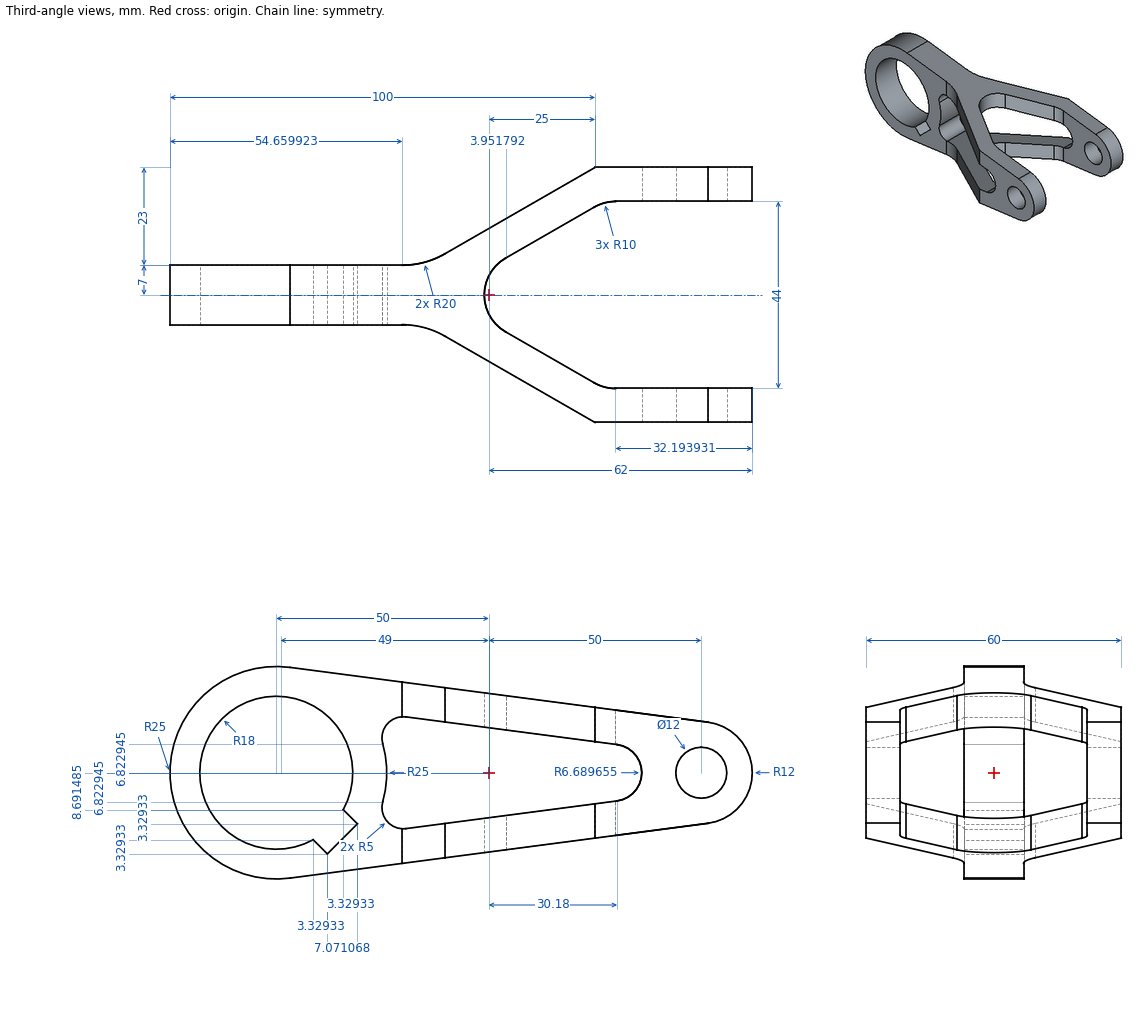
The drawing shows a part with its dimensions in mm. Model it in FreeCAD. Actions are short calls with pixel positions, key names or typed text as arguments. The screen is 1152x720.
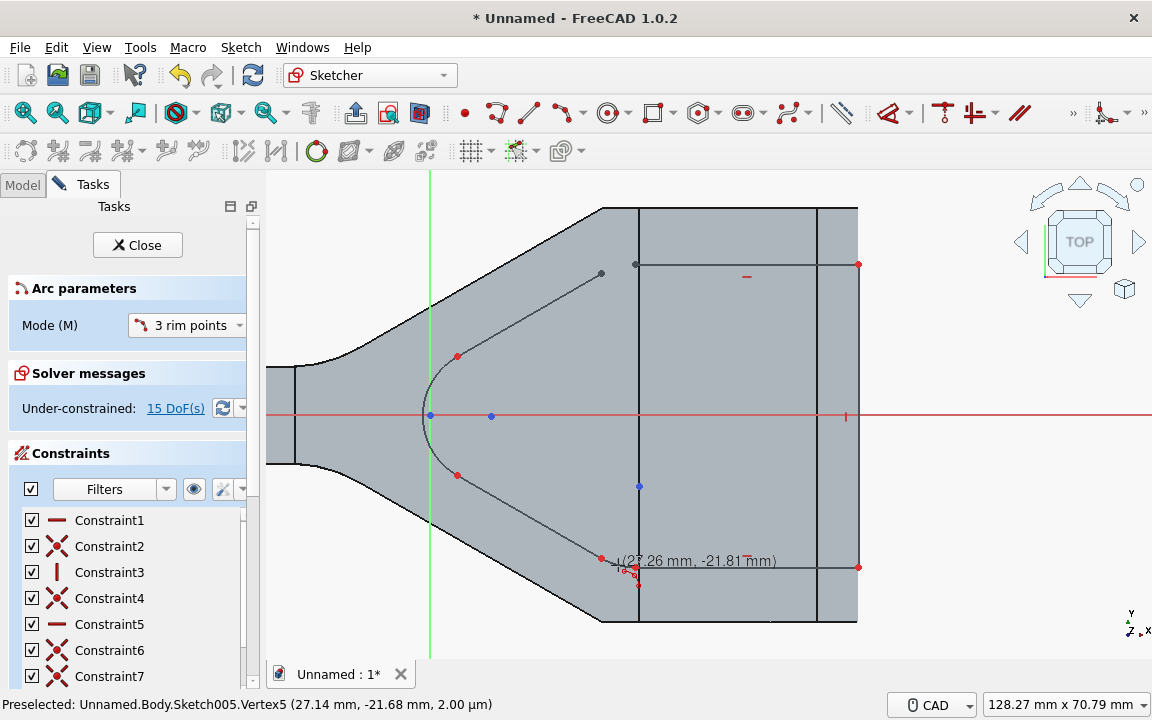
click(636, 265)
click(602, 274)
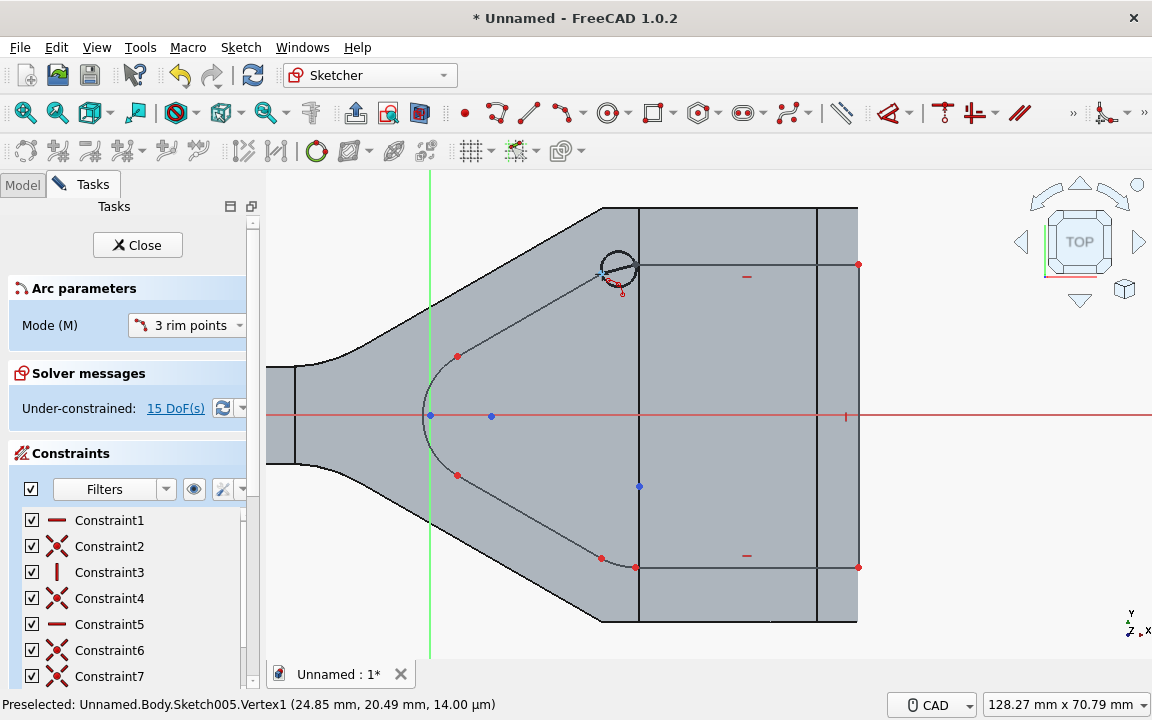
scroll(618, 266, up, 10)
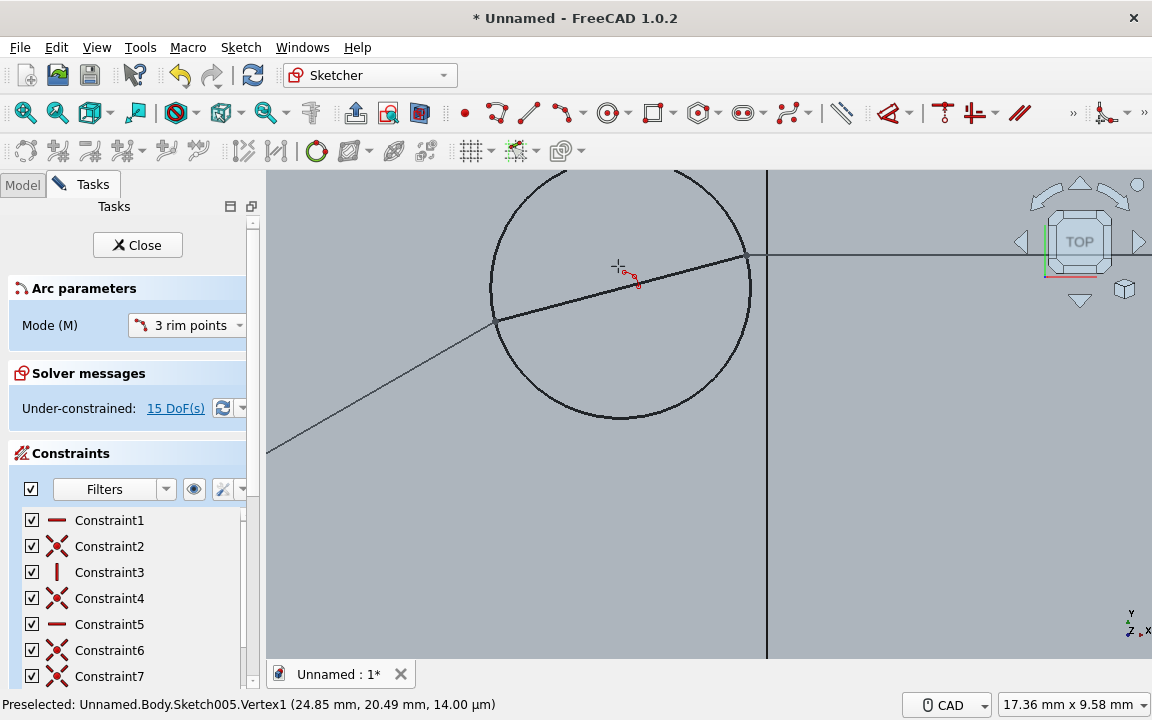
click(616, 262)
key(Escape)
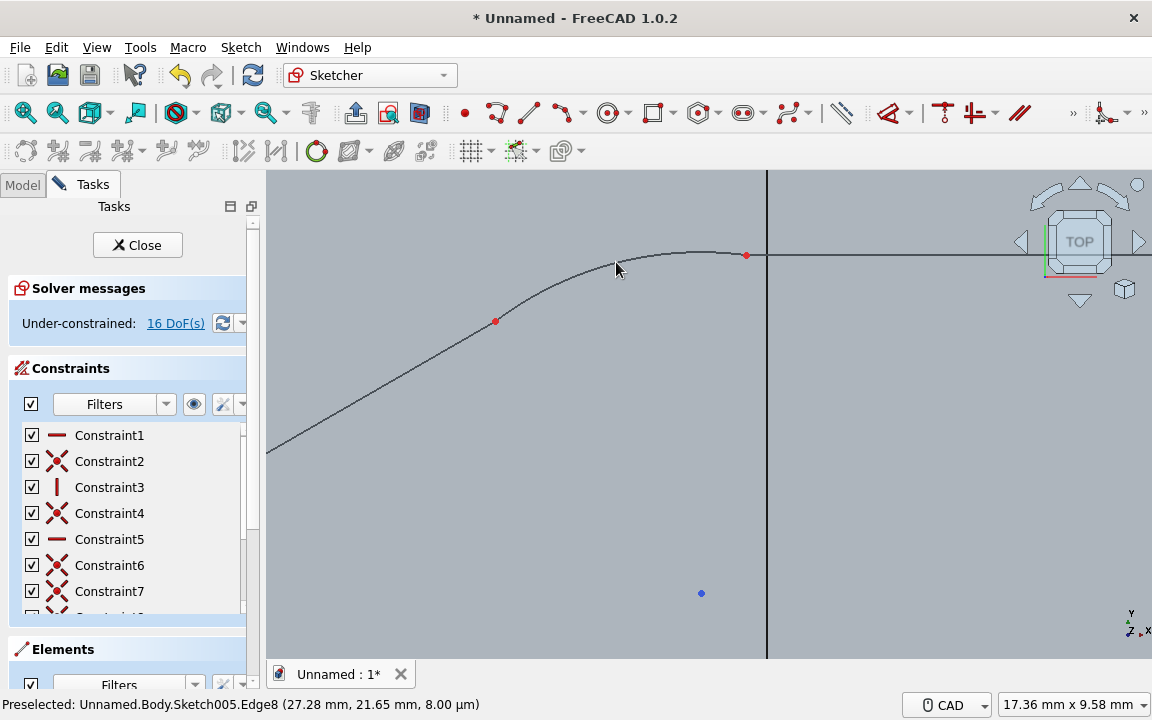
scroll(618, 265, down, 10)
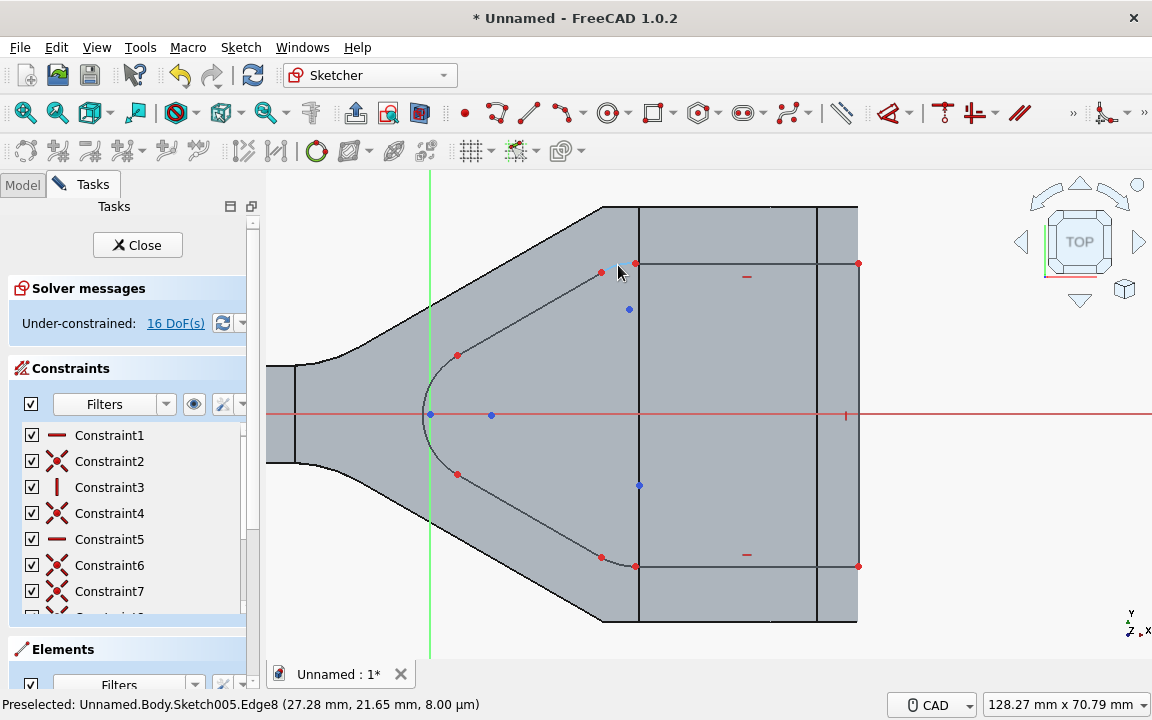
click(558, 298)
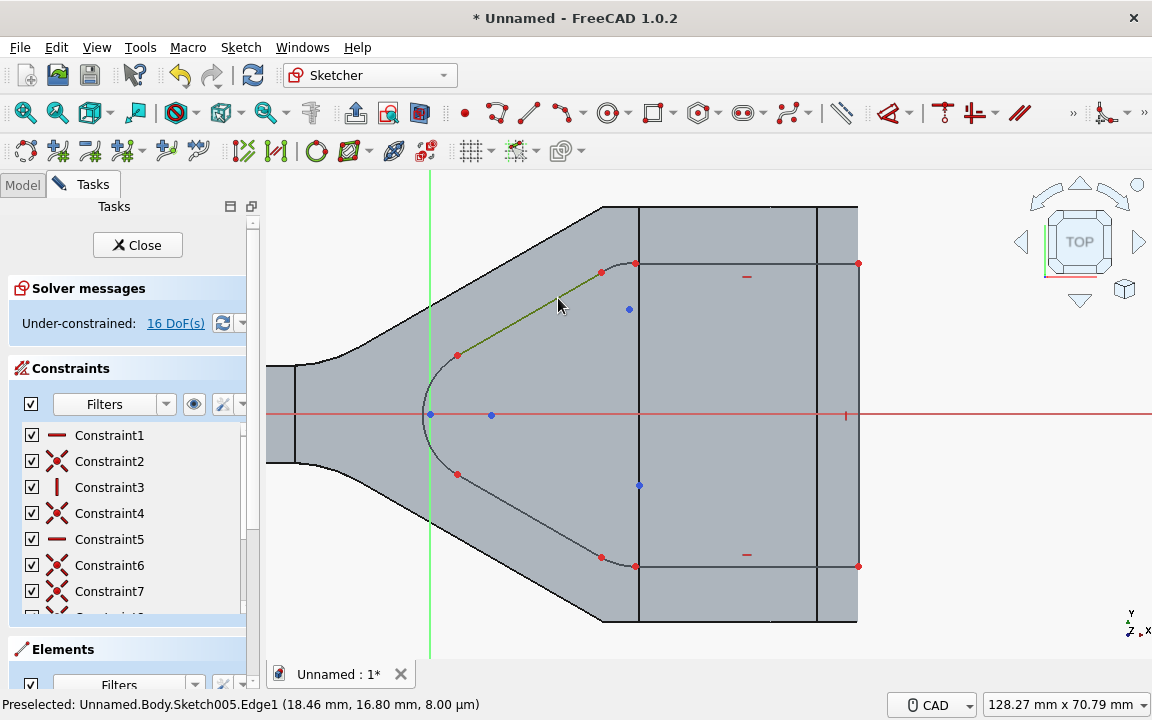
click(429, 387)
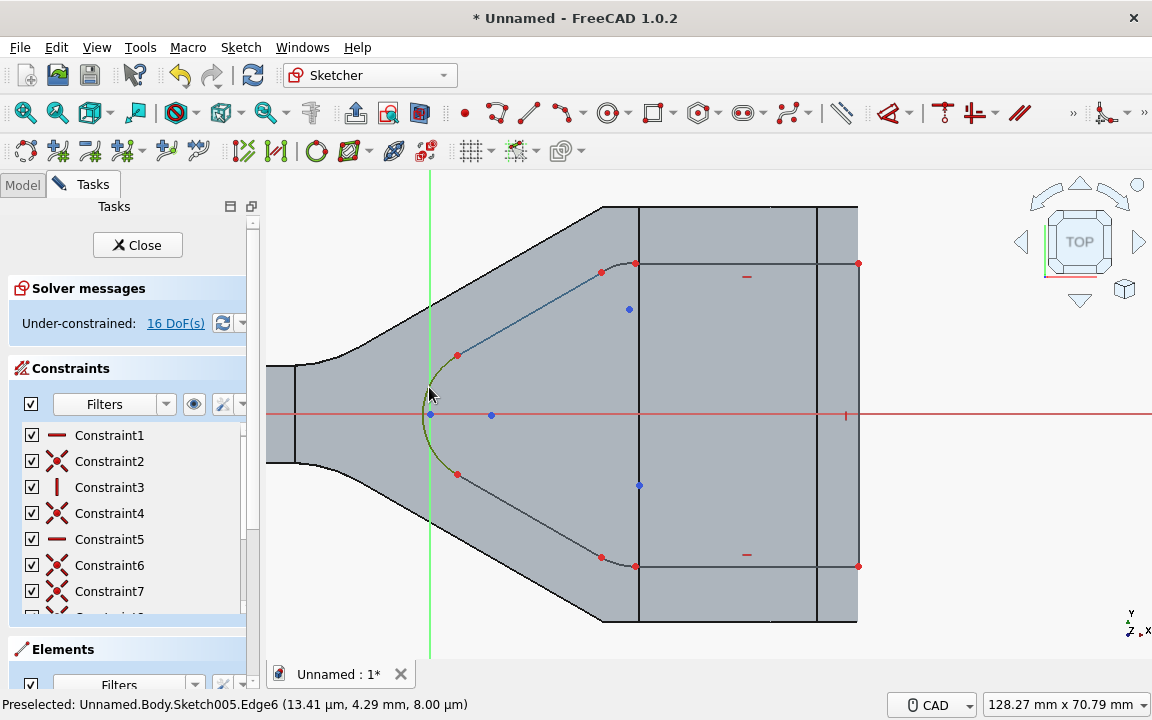
key(t)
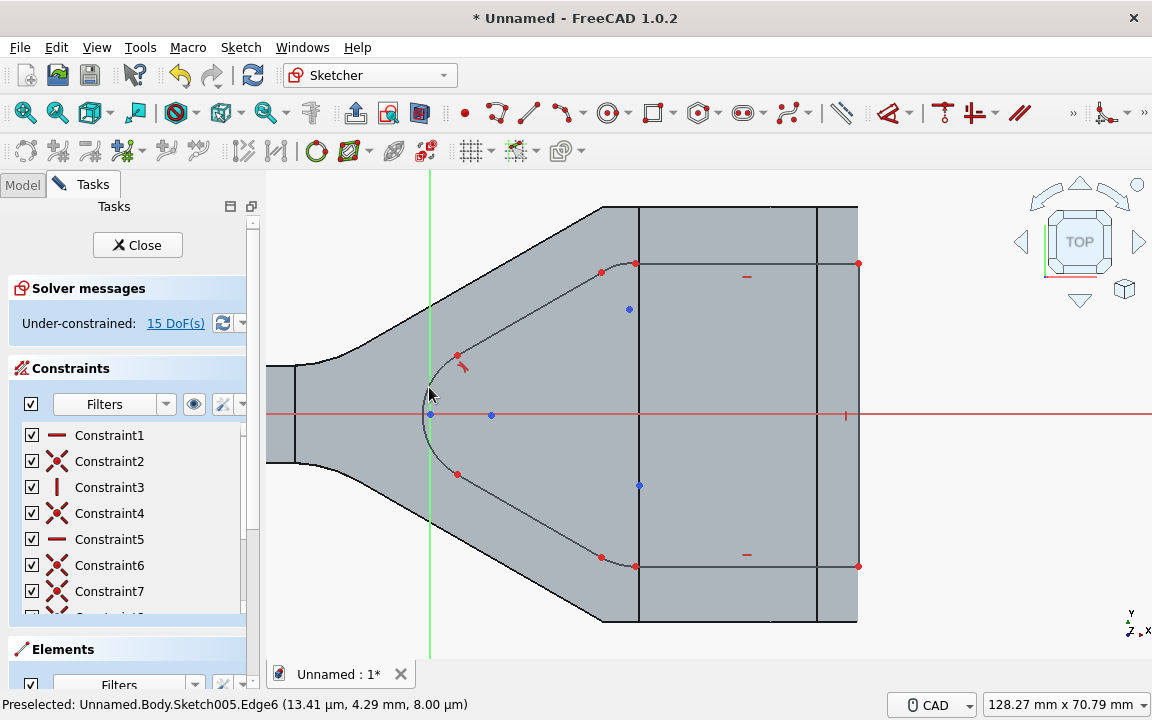
click(558, 298)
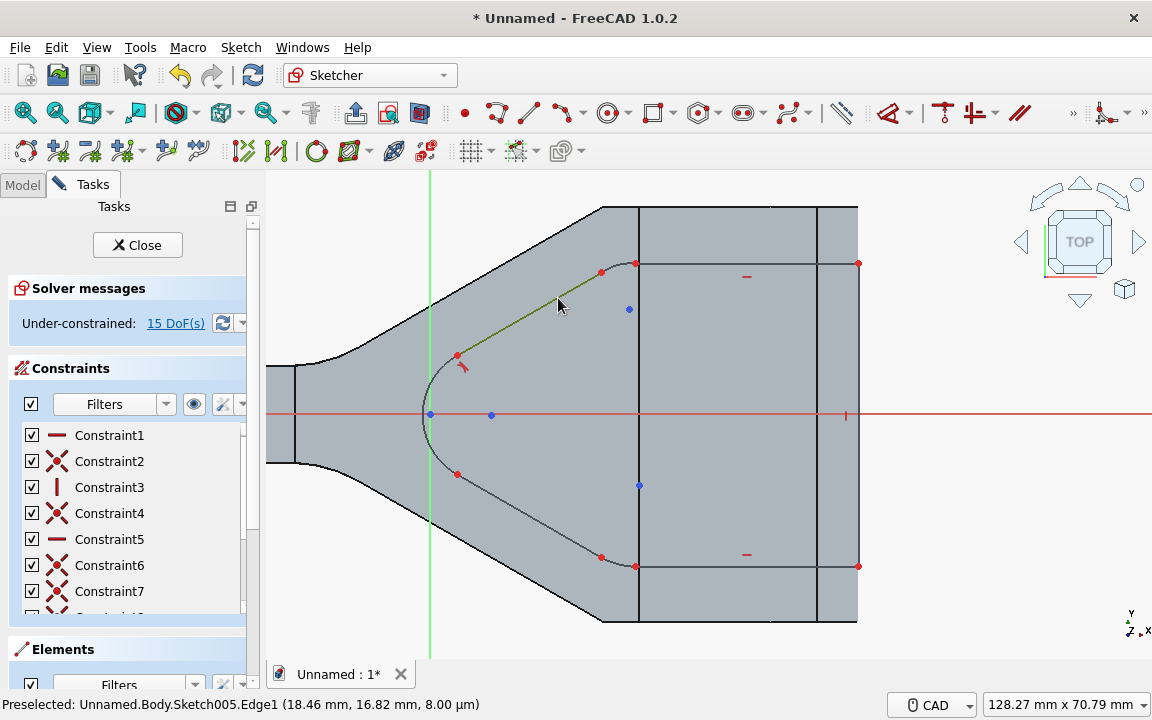
scroll(625, 264, up, 2)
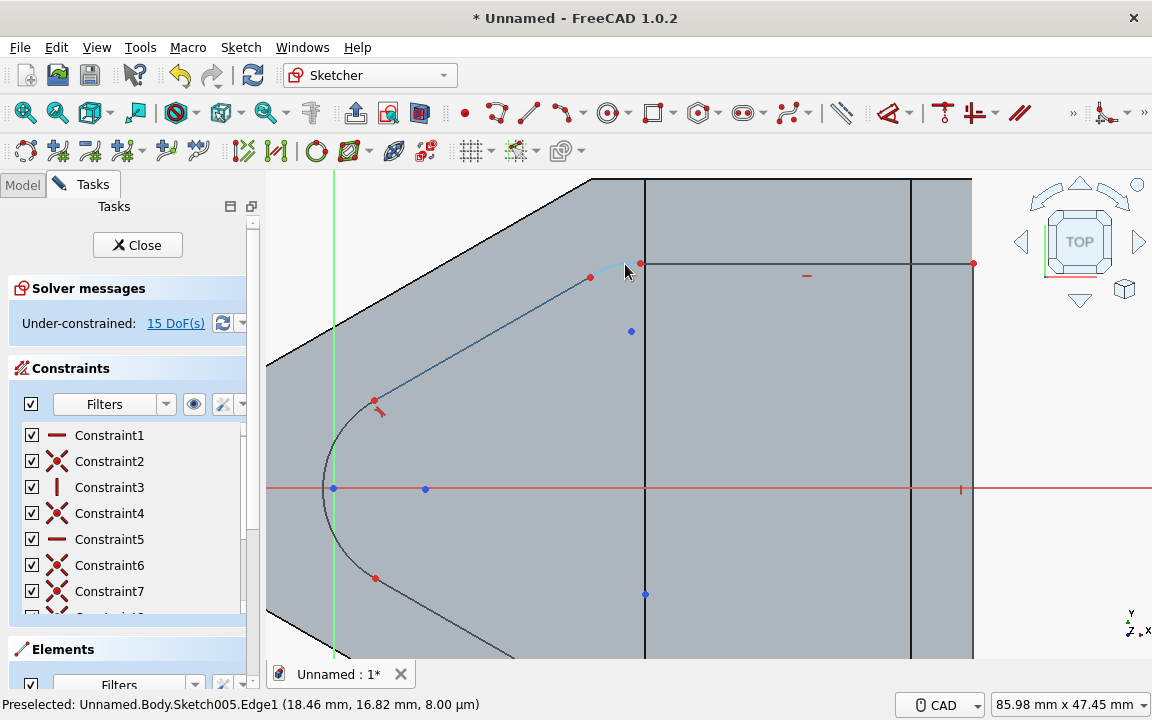
click(625, 263)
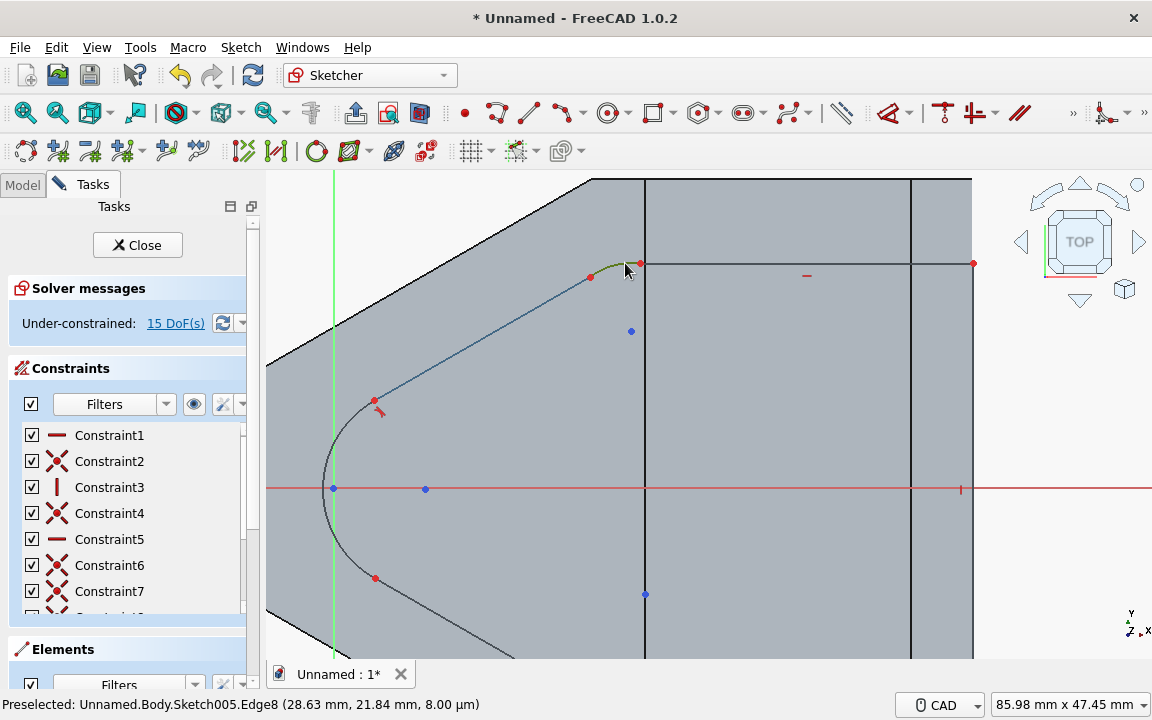
key(t)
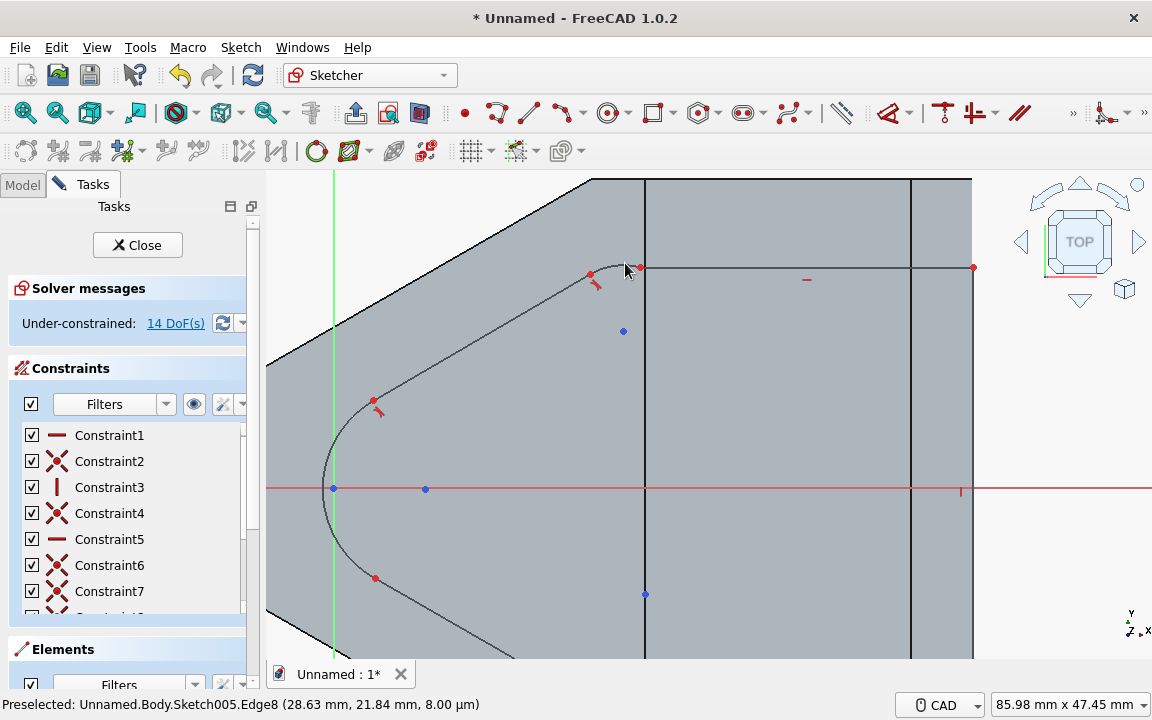
click(440, 616)